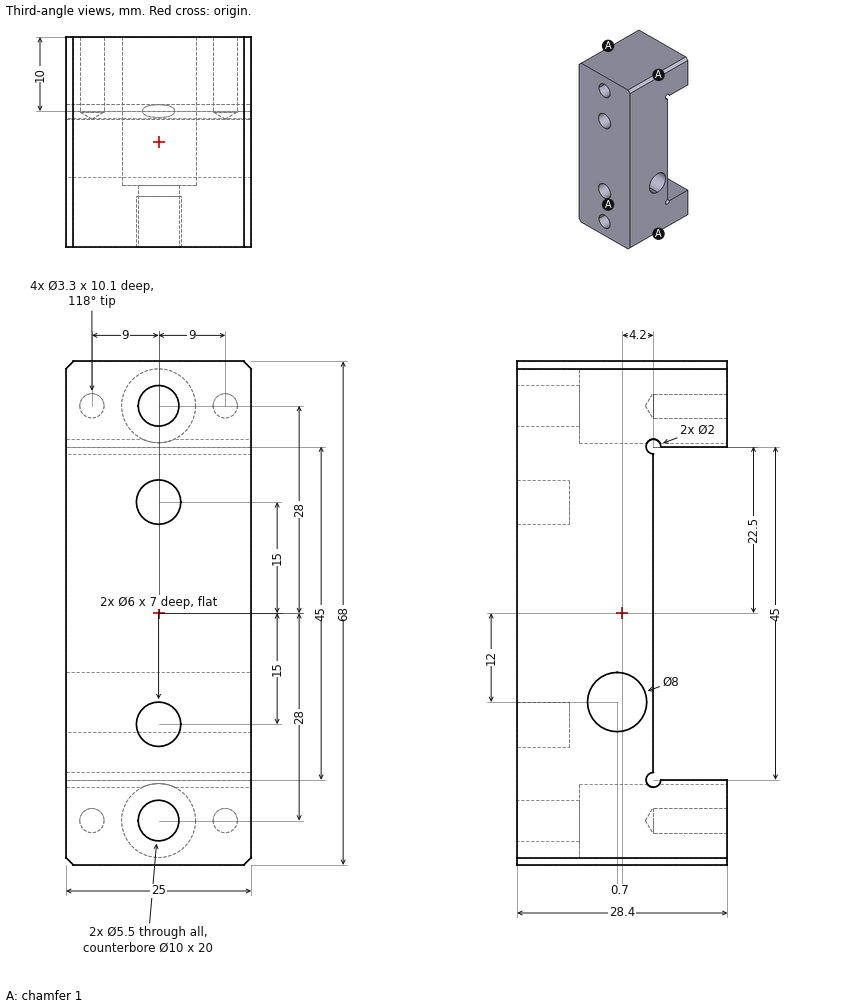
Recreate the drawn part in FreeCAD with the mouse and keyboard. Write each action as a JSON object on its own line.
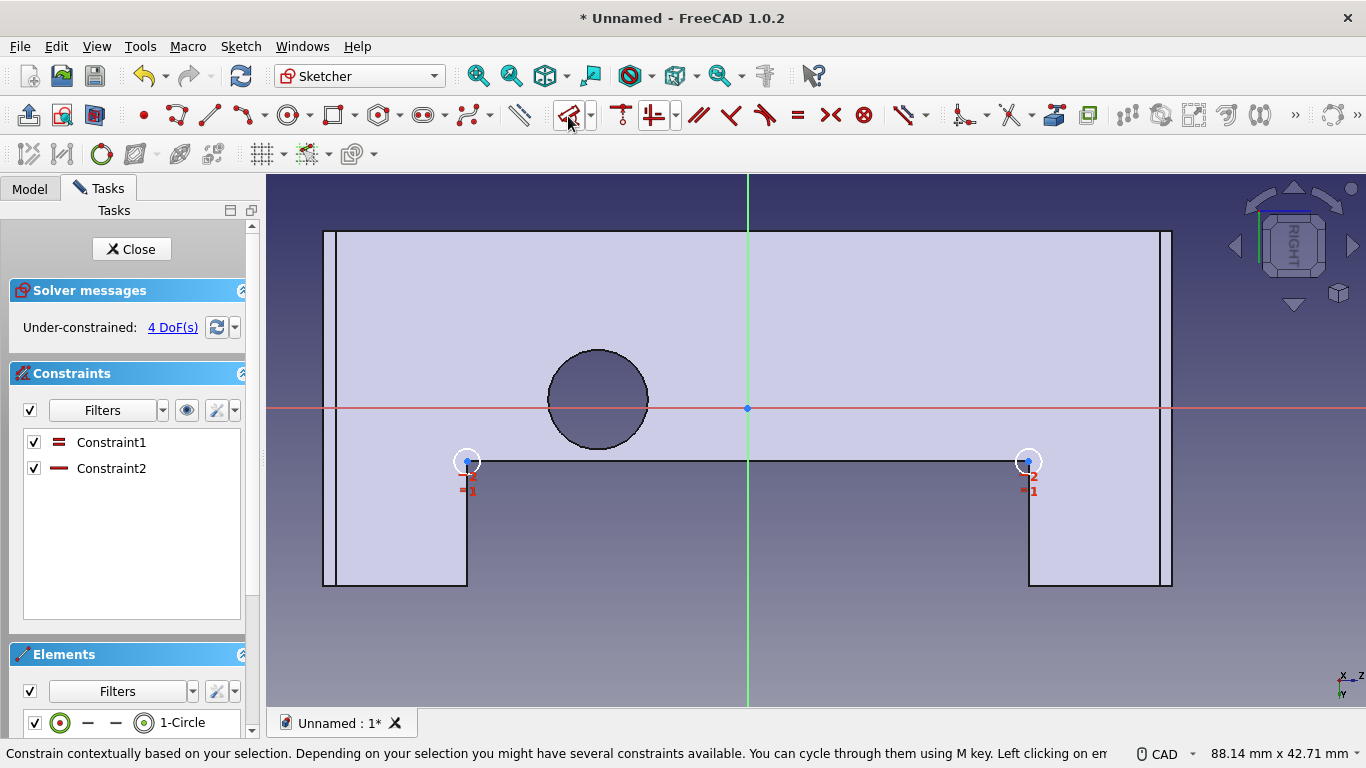
{"action": "scroll", "coordinate": [1038, 453], "scroll_direction": "up", "scroll_amount": 3}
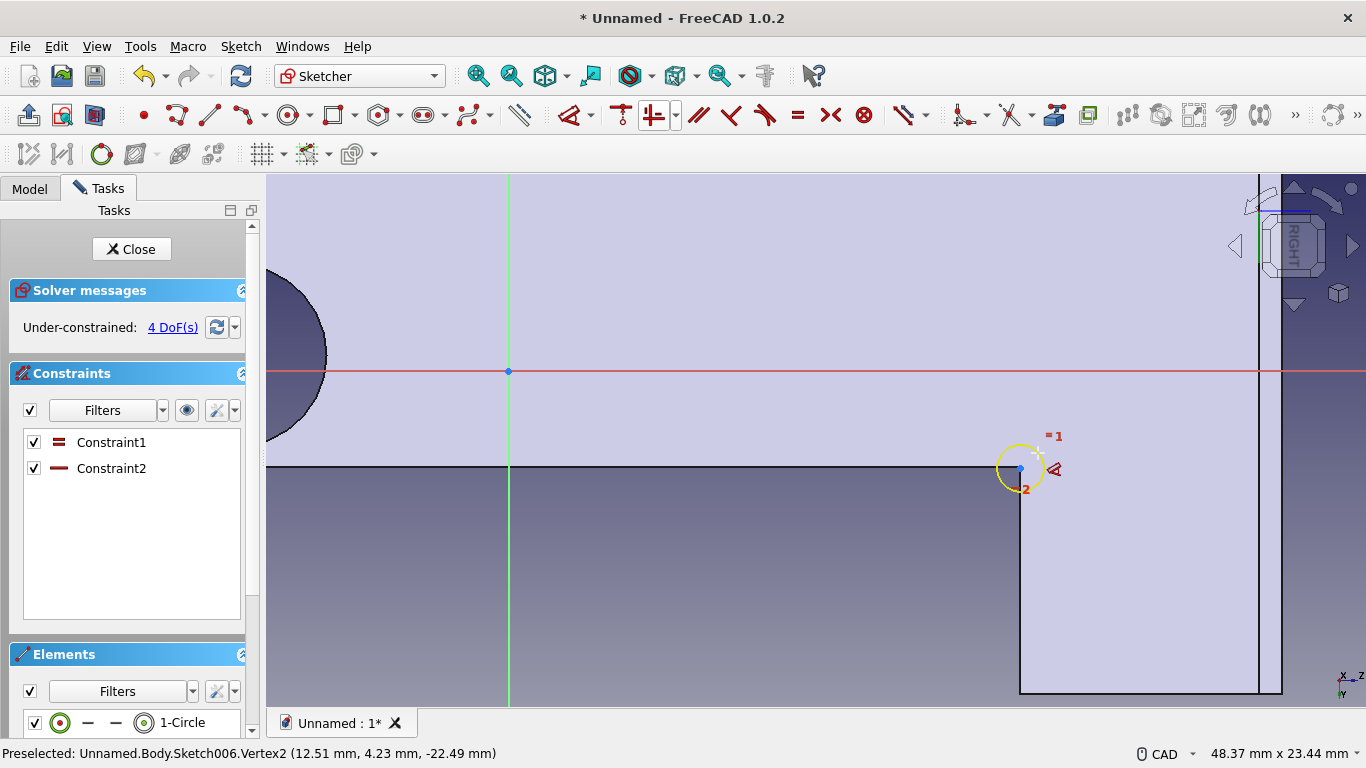
{"action": "left_click", "coordinate": [1037, 452]}
{"action": "left_click", "coordinate": [1060, 429]}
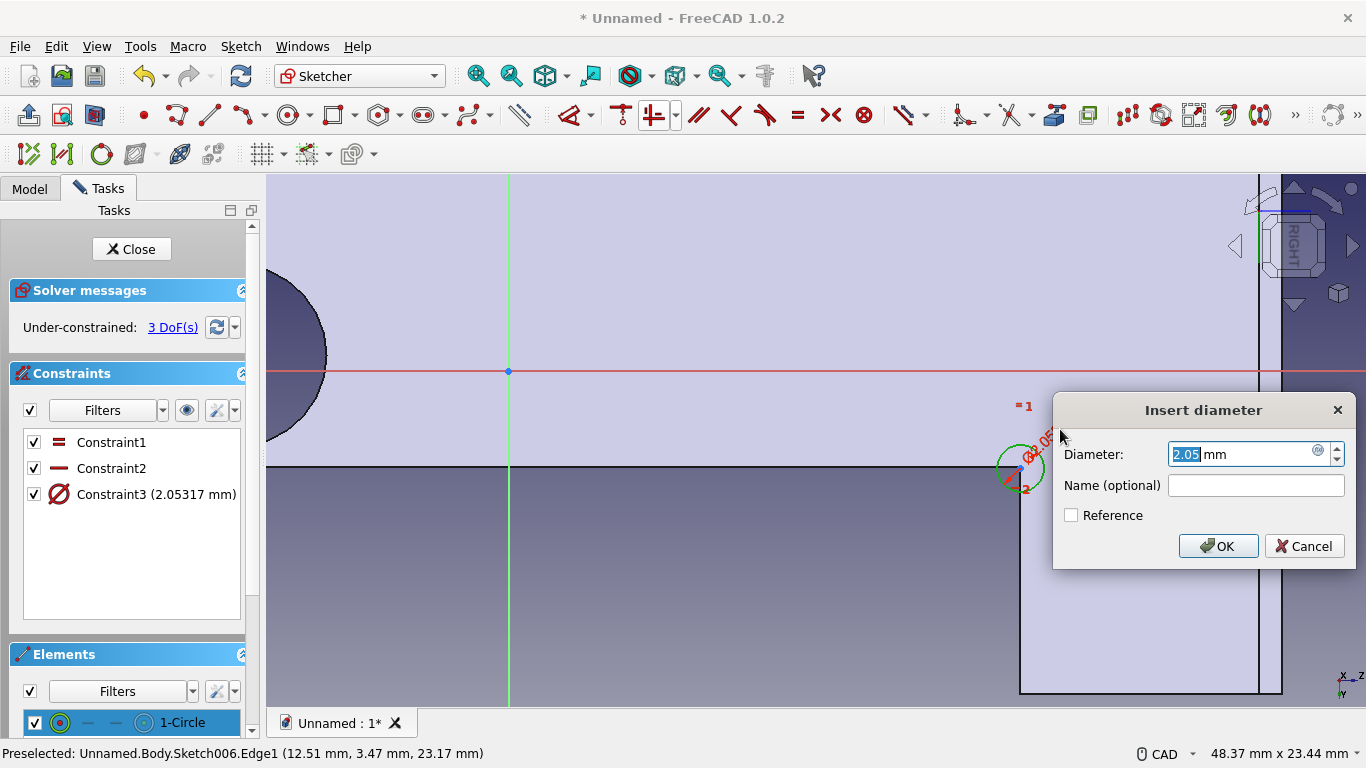
{"action": "type", "text": "2"}
{"action": "key", "text": "Return"}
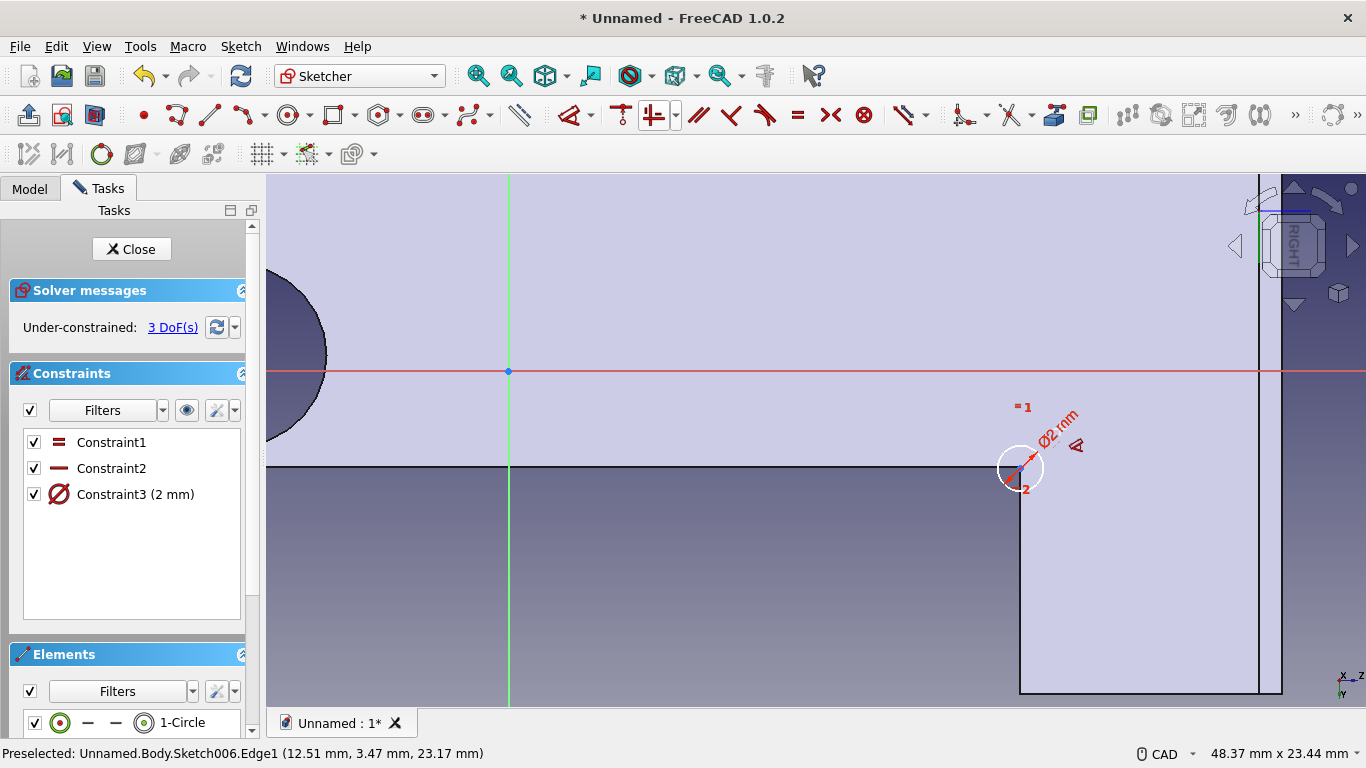
{"action": "left_click", "coordinate": [1021, 468]}
{"action": "left_click", "coordinate": [1055, 398]}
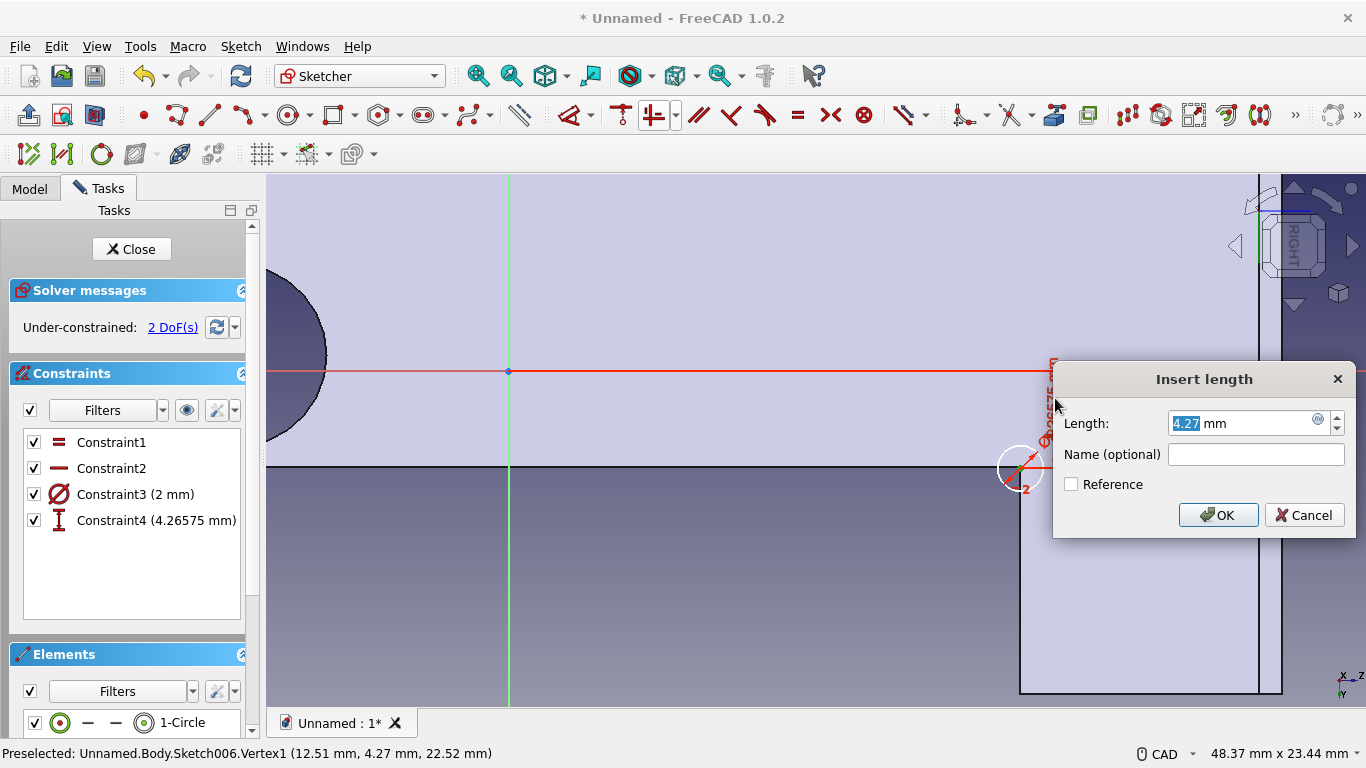
{"action": "type", "text": "4.2"}
{"action": "key", "text": "Return"}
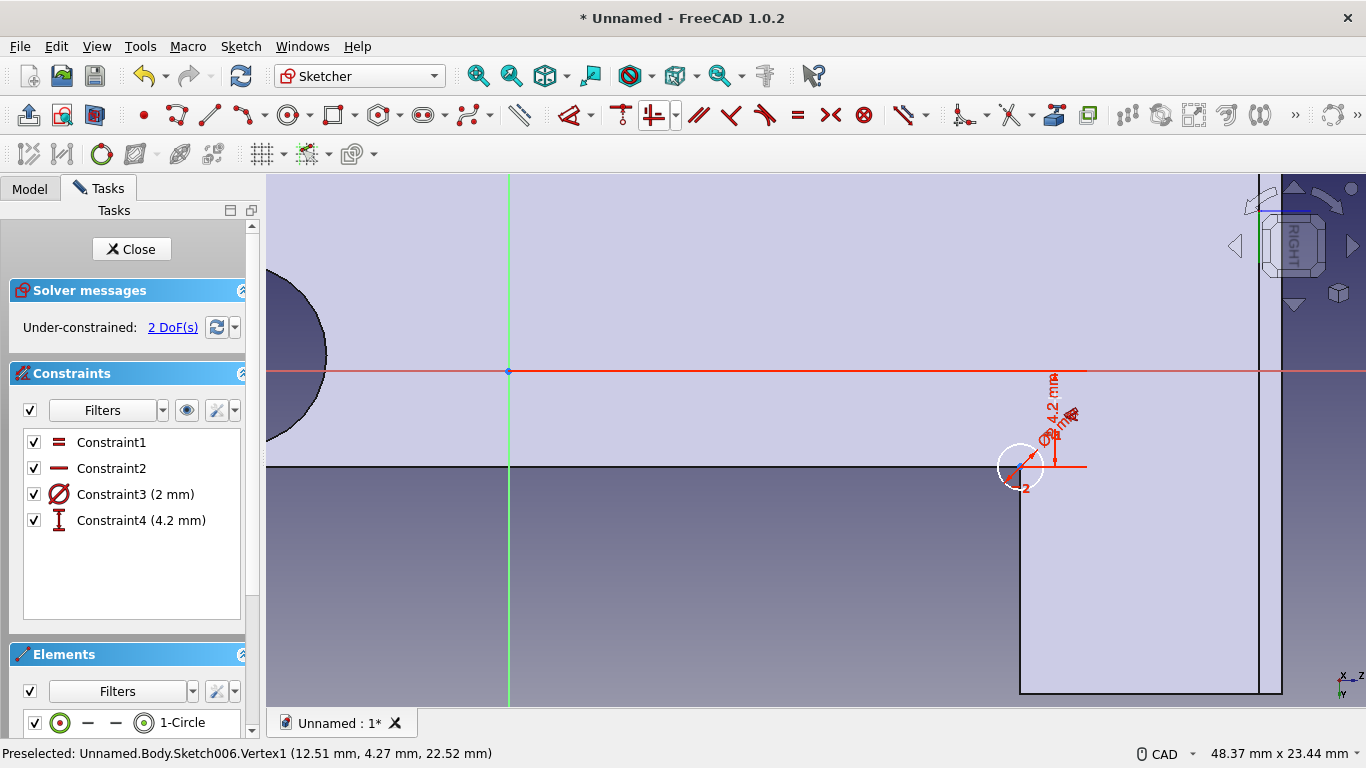
{"action": "left_click", "coordinate": [1021, 467]}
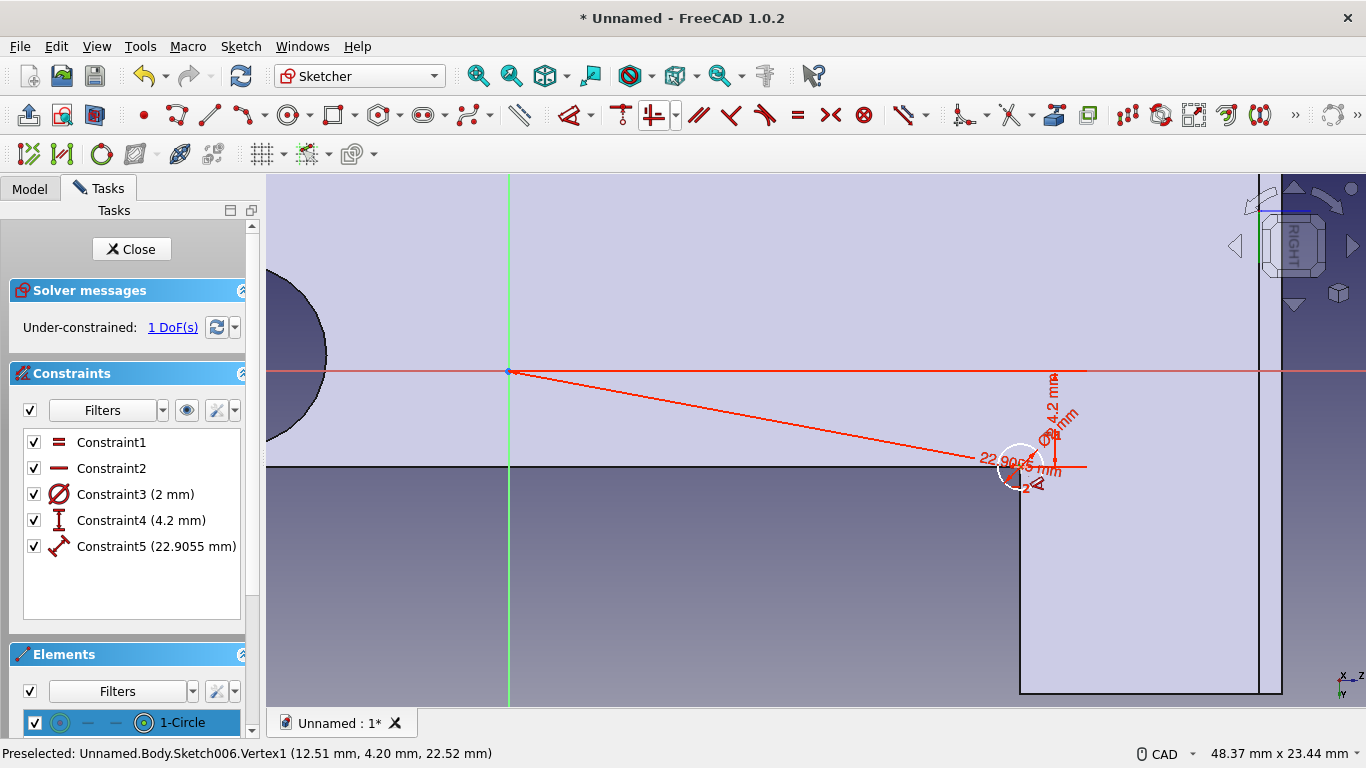
{"action": "scroll", "coordinate": [1038, 453], "scroll_direction": "down", "scroll_amount": 3}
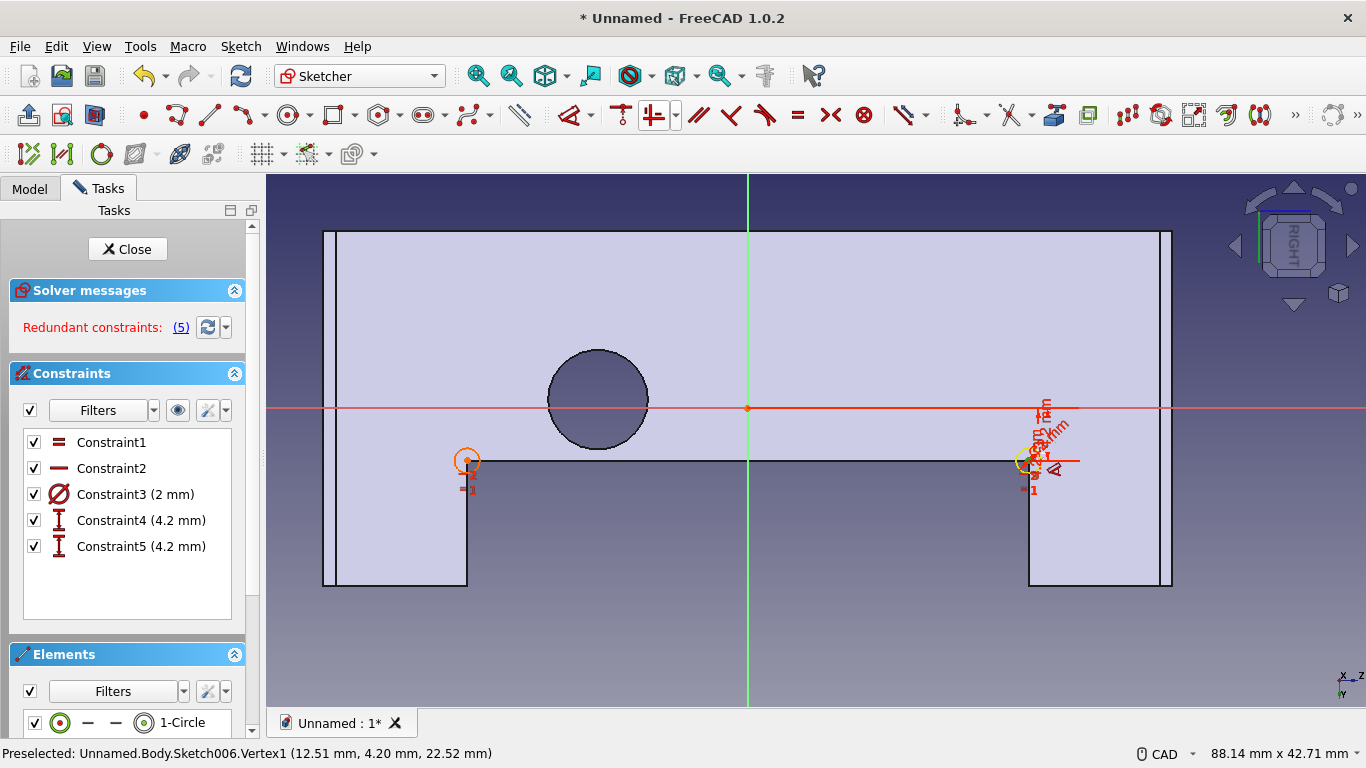
{"action": "left_click", "coordinate": [467, 461]}
{"action": "left_click", "coordinate": [619, 495]}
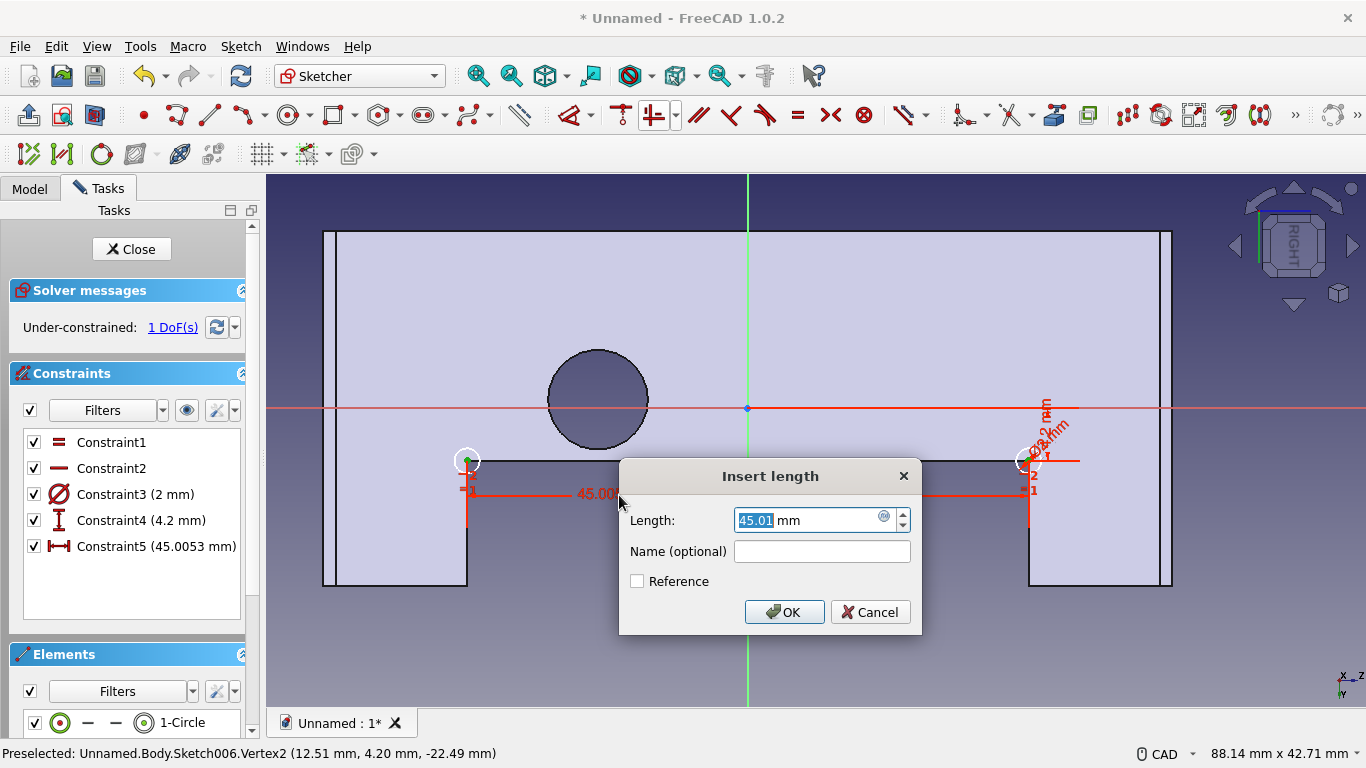
{"action": "type", "text": "45"}
{"action": "key", "text": "Return"}